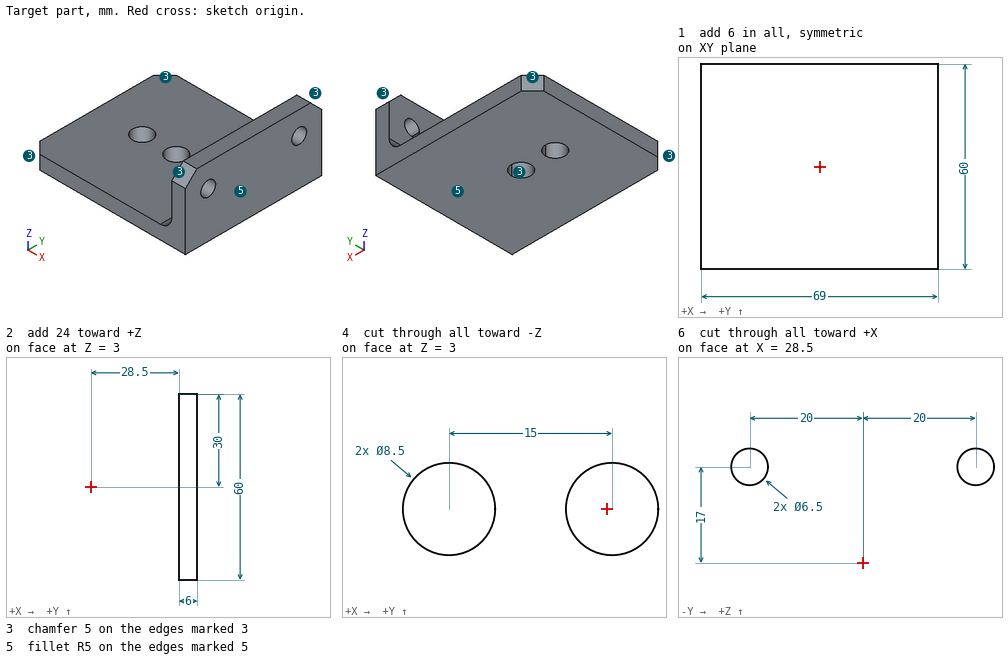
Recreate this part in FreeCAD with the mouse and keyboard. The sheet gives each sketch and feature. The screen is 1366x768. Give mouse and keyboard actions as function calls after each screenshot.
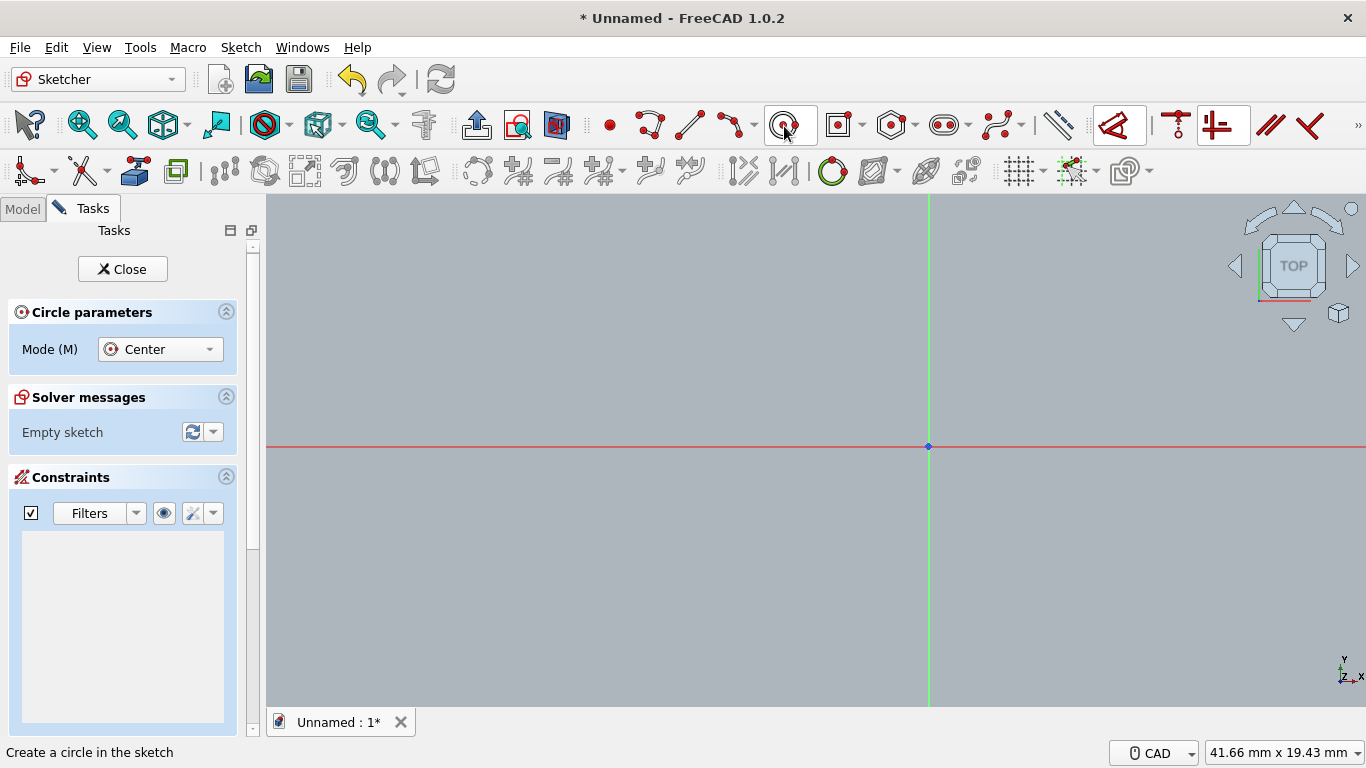
click(546, 447)
move(625, 367)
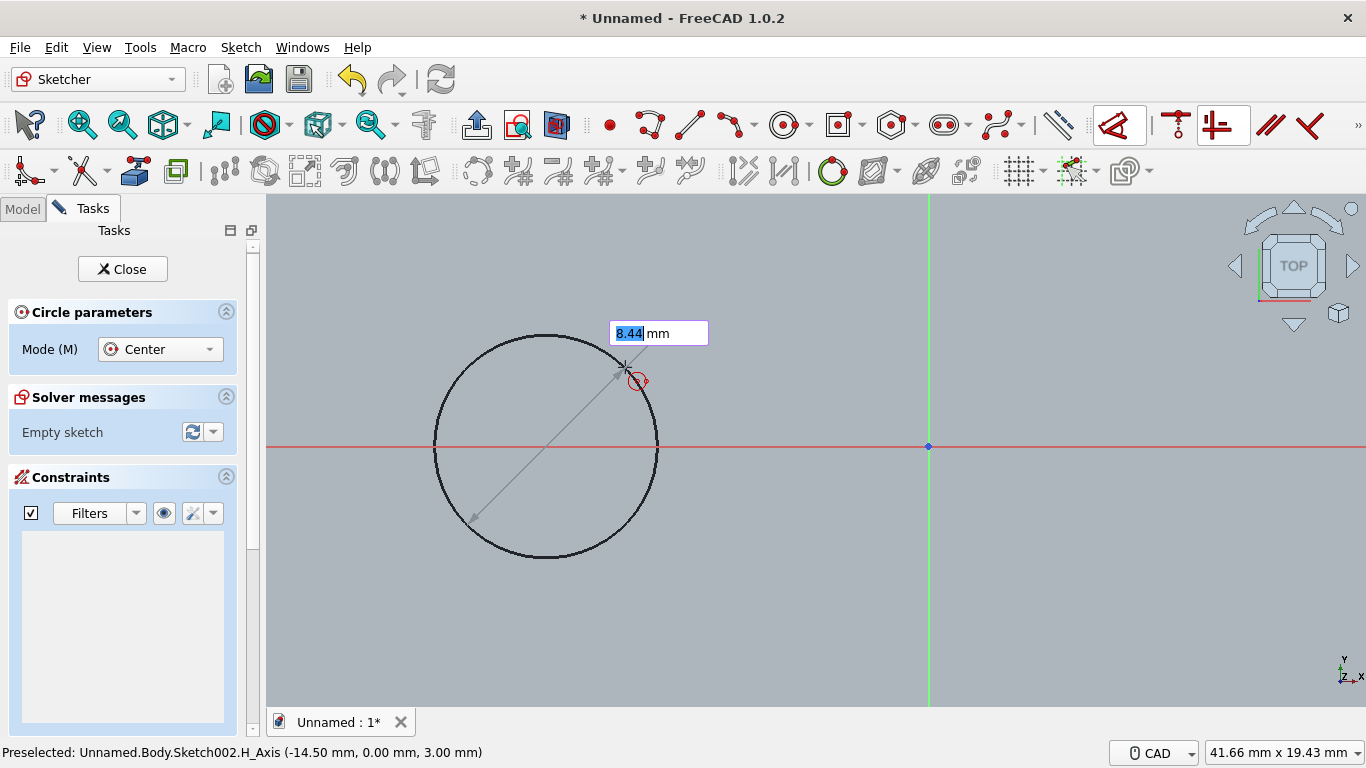
text(8.5)
key(Return)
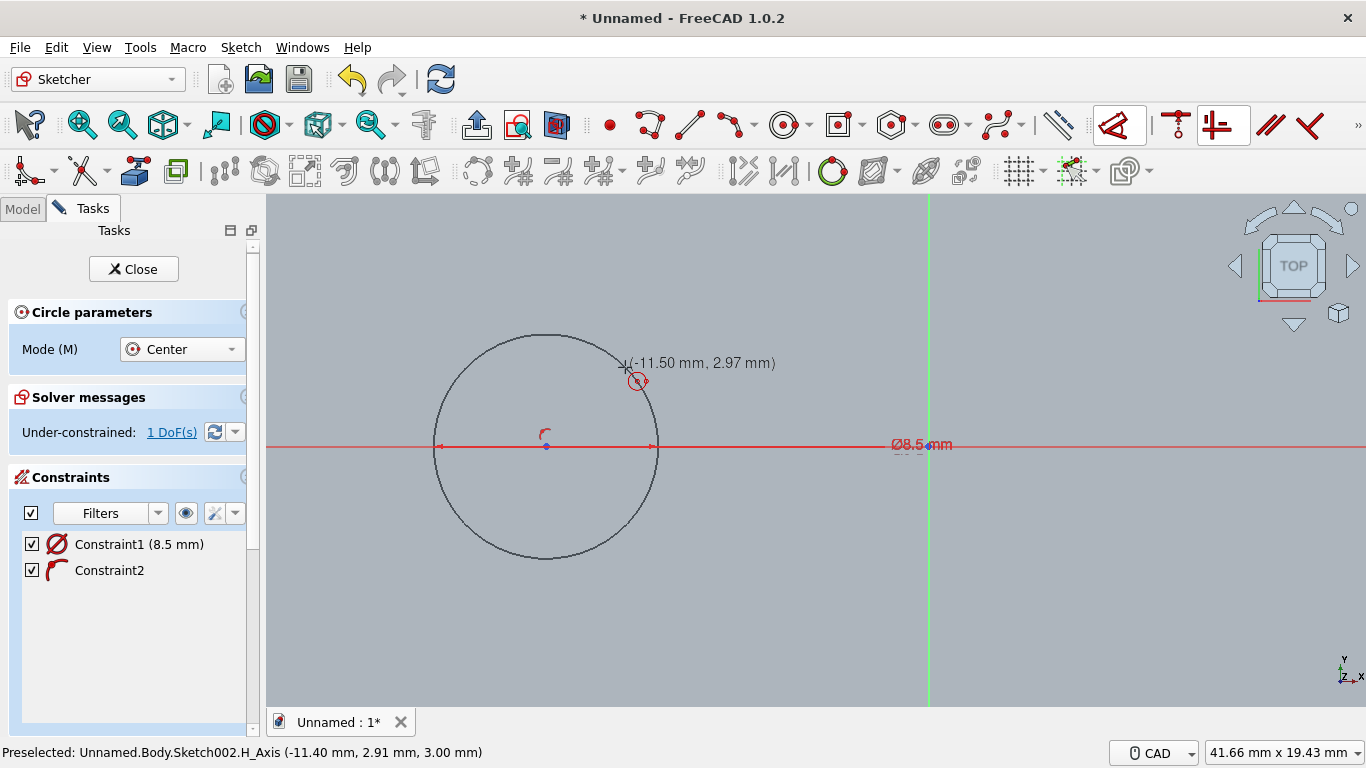
click(942, 447)
move(1021, 367)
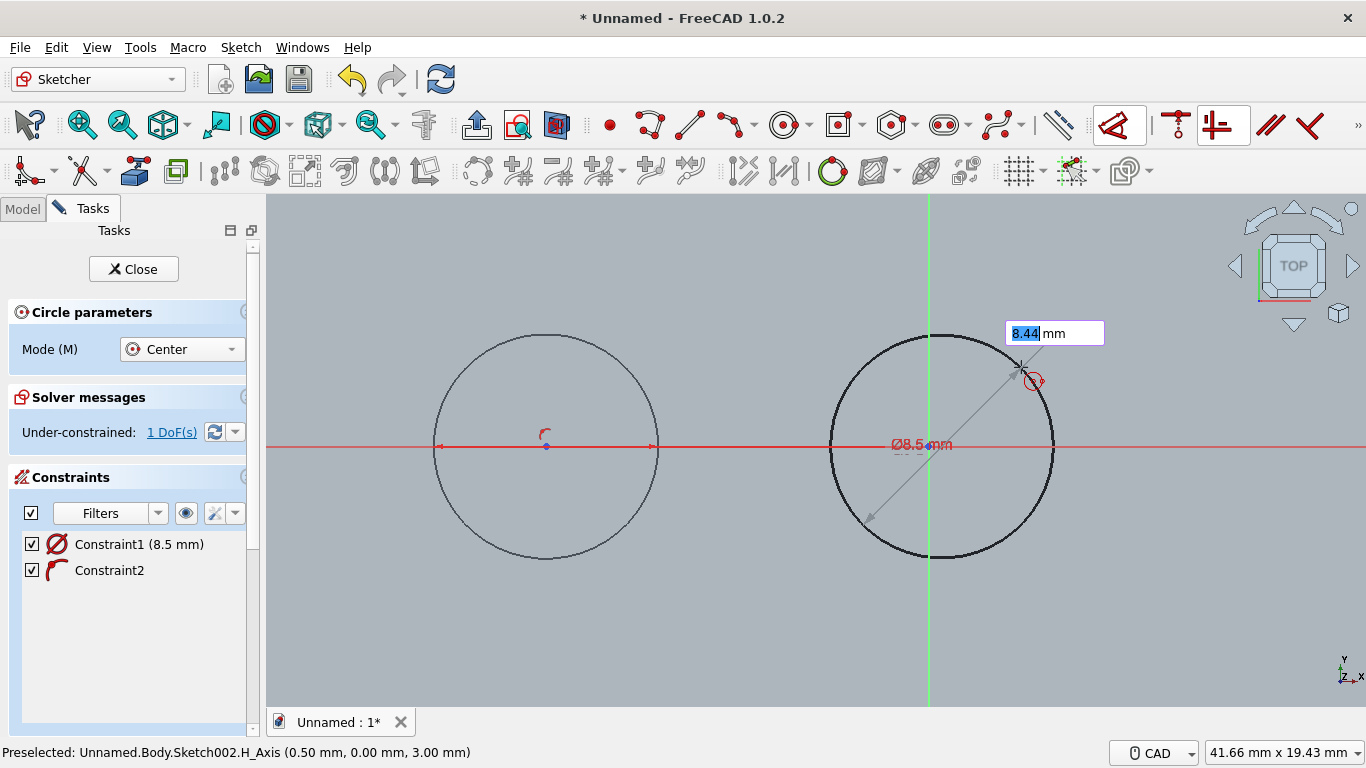
text(8.5)
key(Return)
key(Escape)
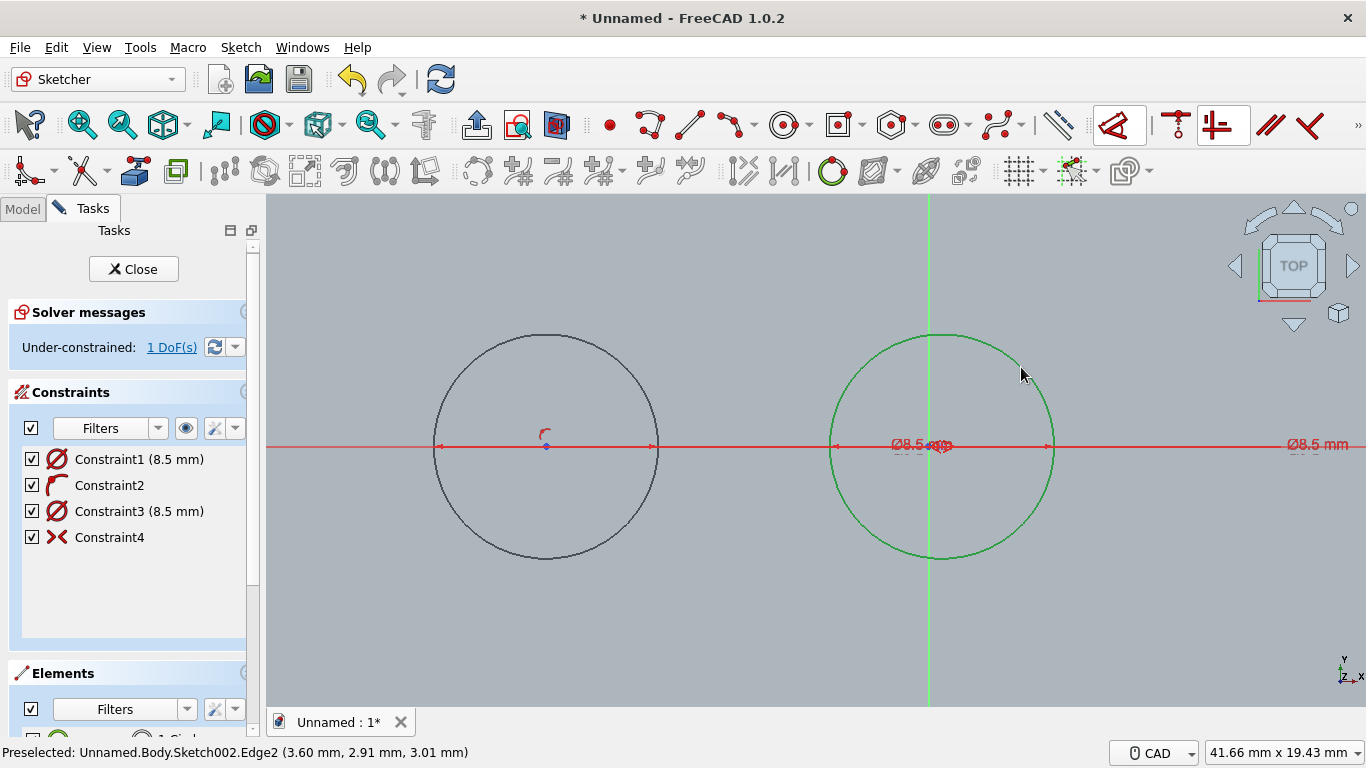
click(546, 447)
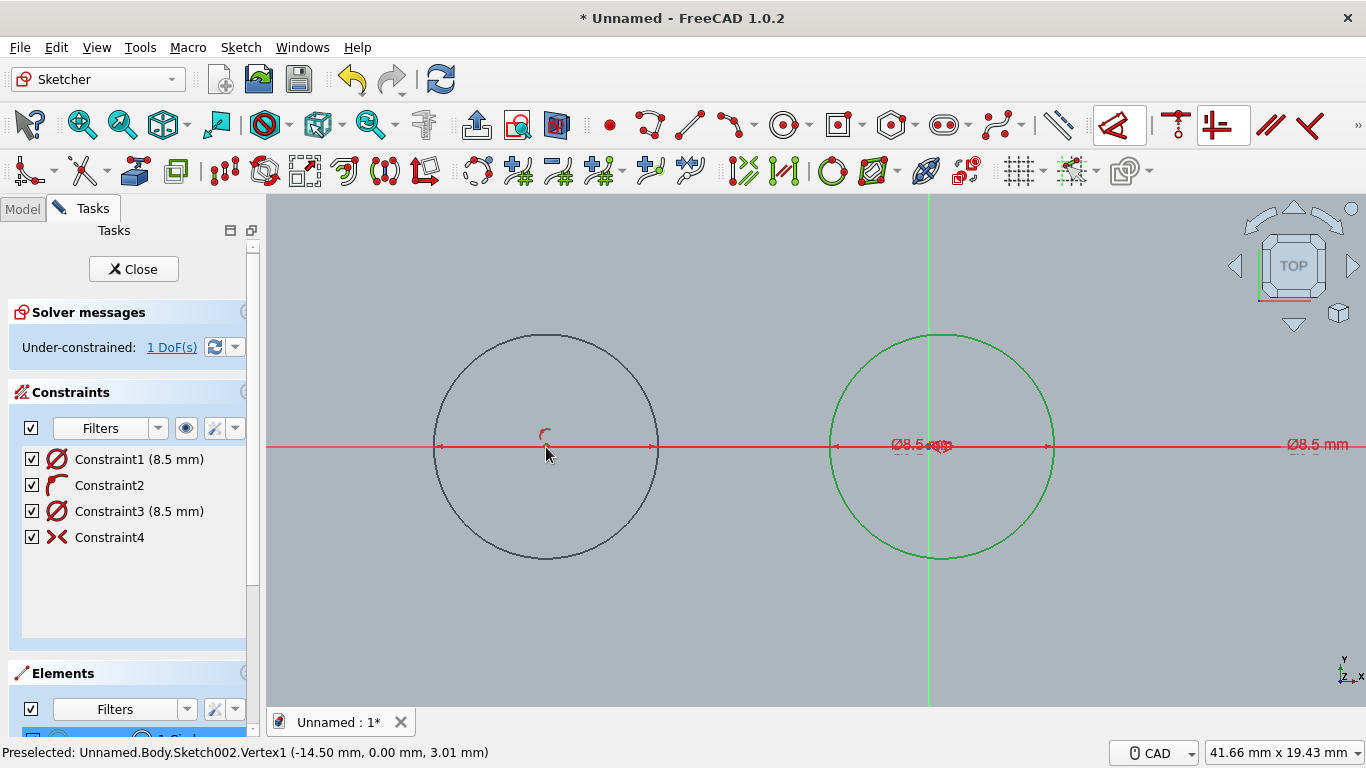
click(942, 447)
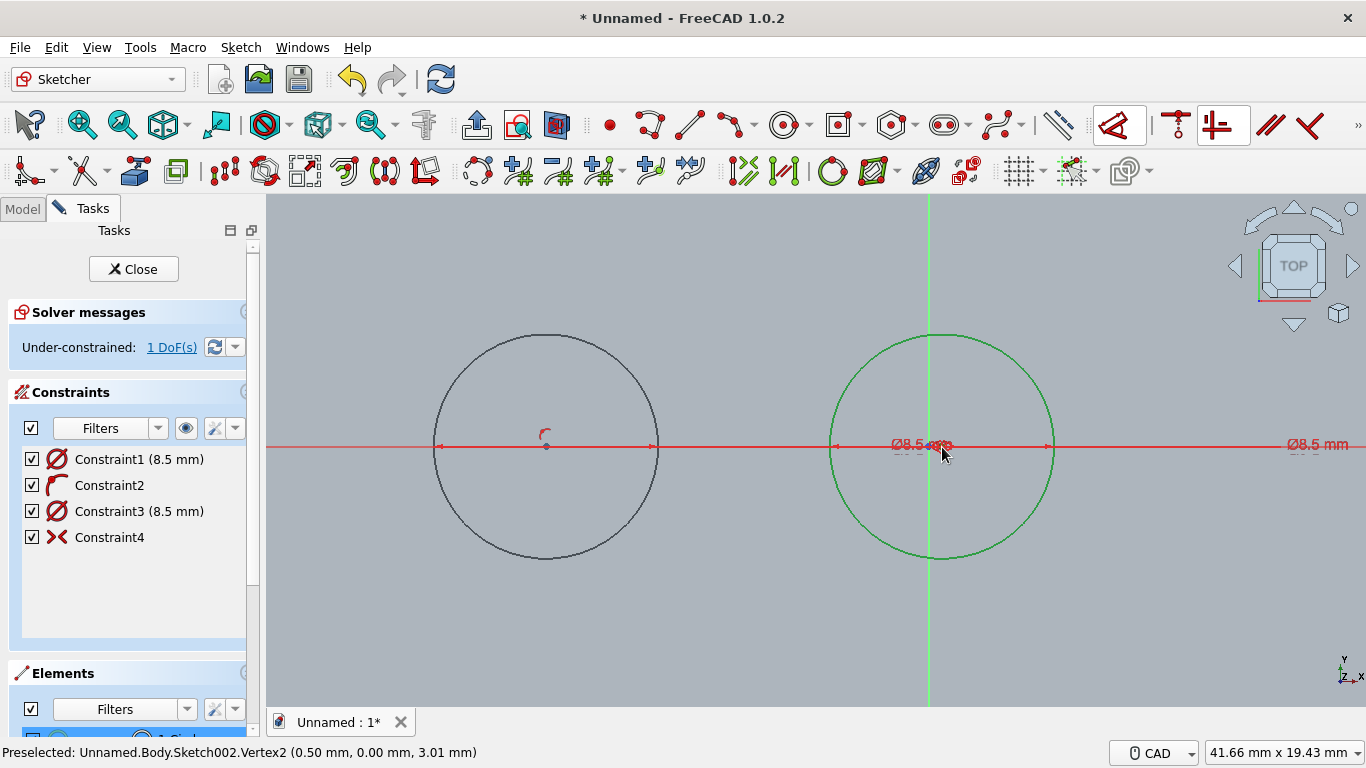
key(l)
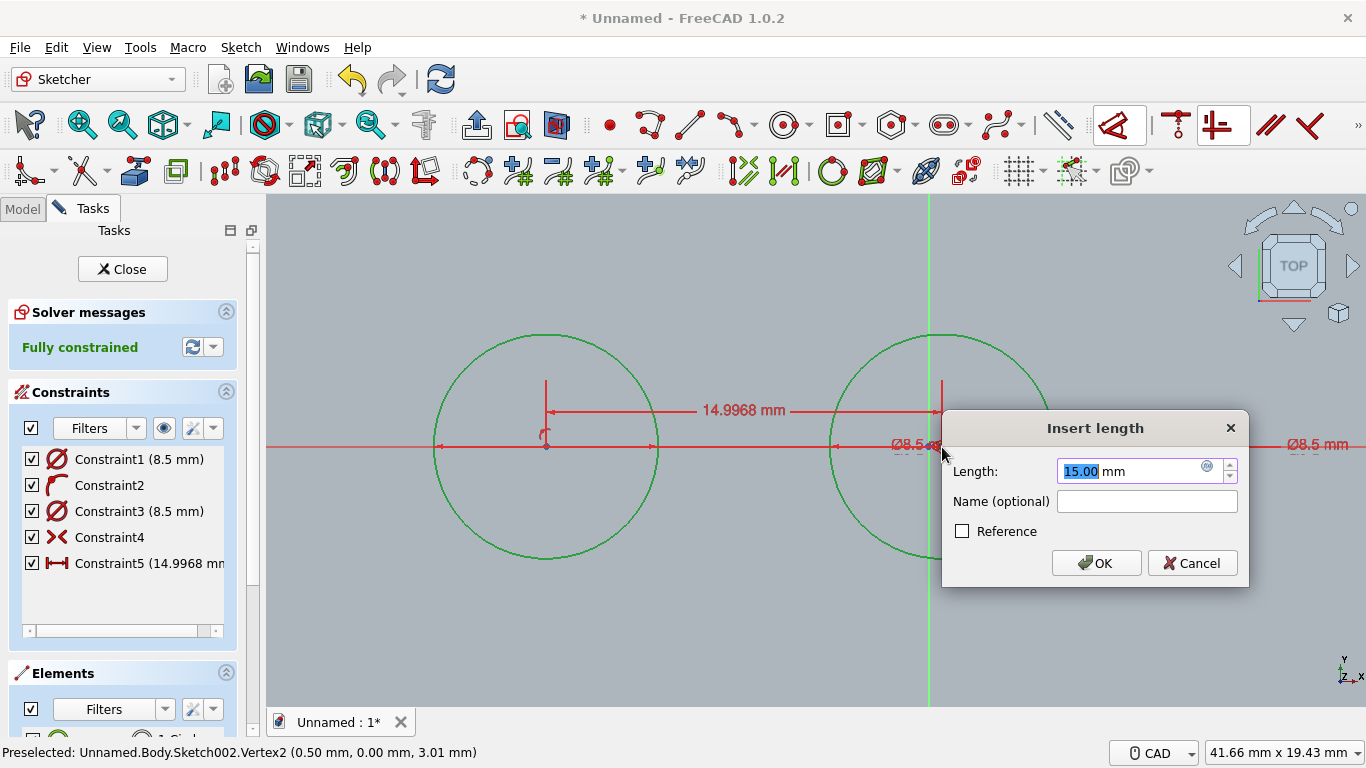
text(15)
key(Return)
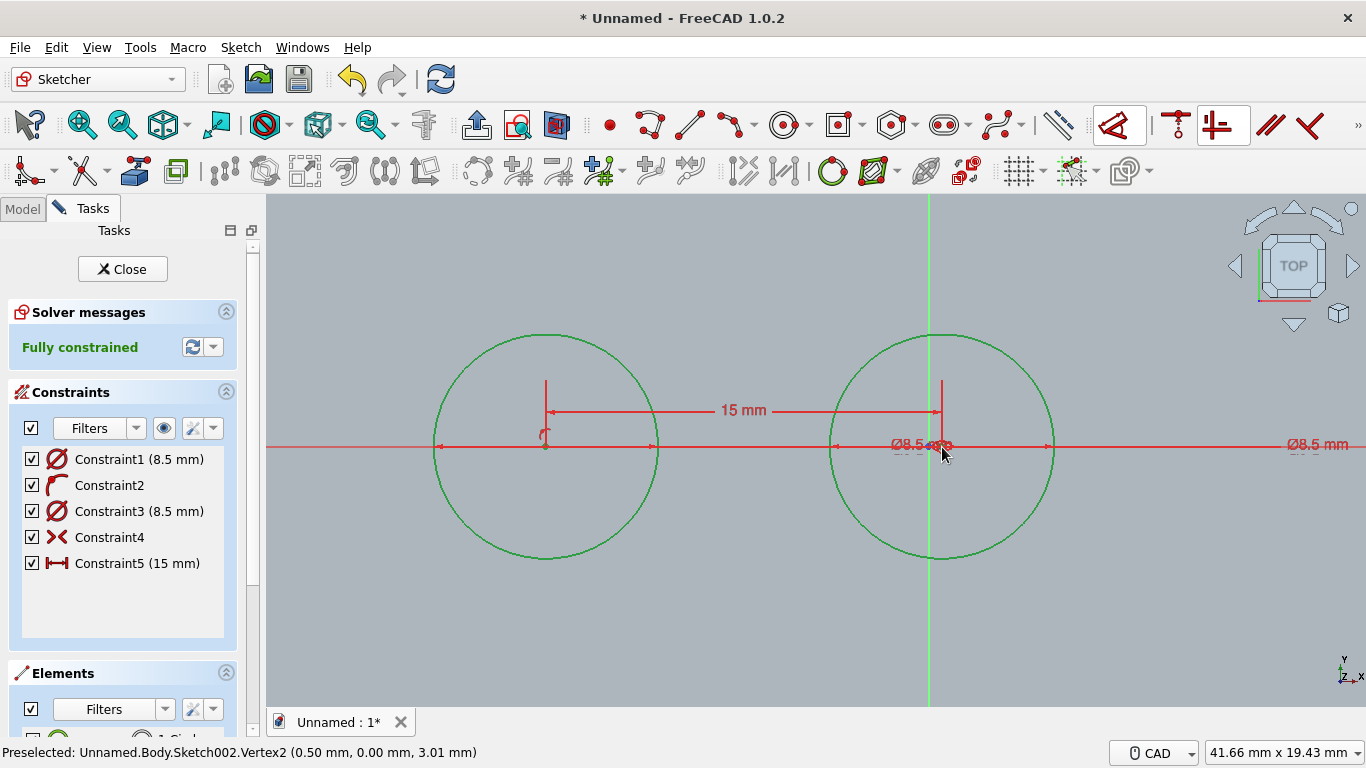
click(123, 269)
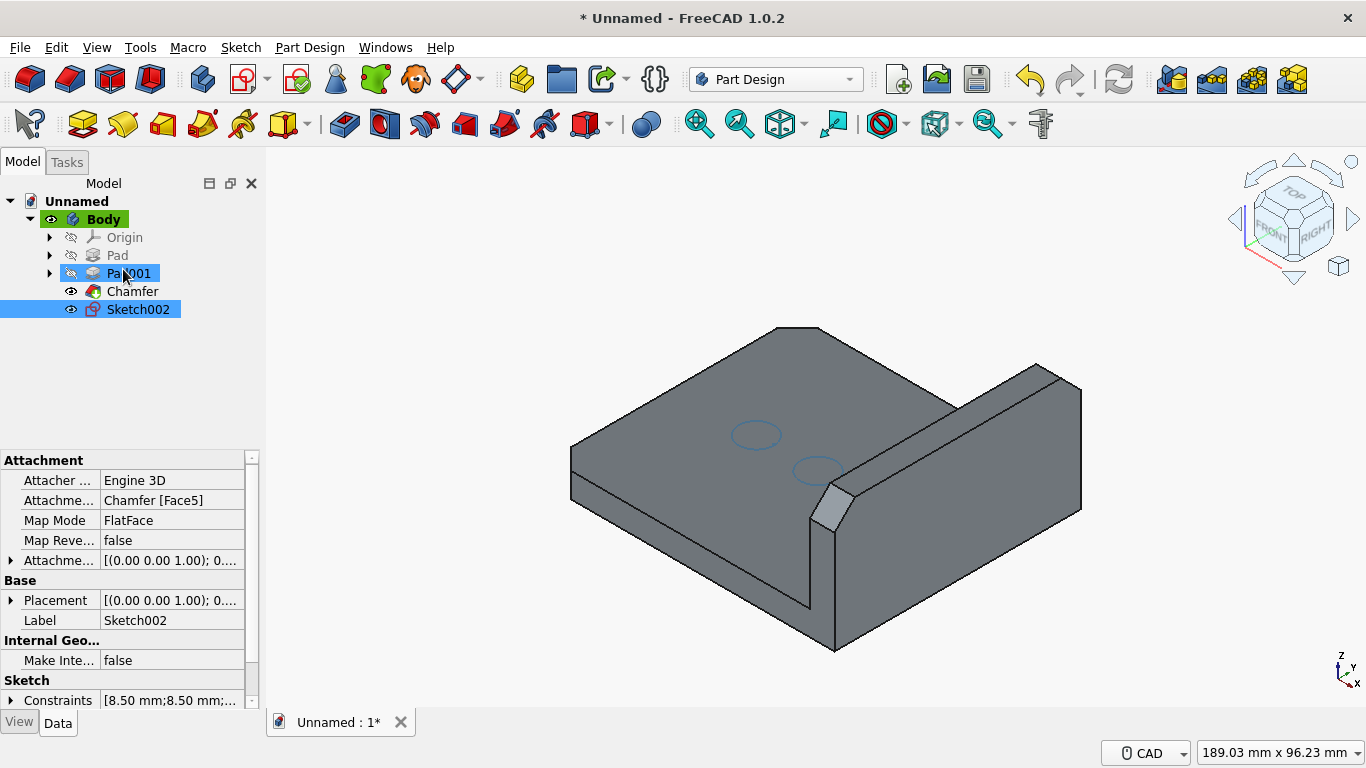
click(346, 124)